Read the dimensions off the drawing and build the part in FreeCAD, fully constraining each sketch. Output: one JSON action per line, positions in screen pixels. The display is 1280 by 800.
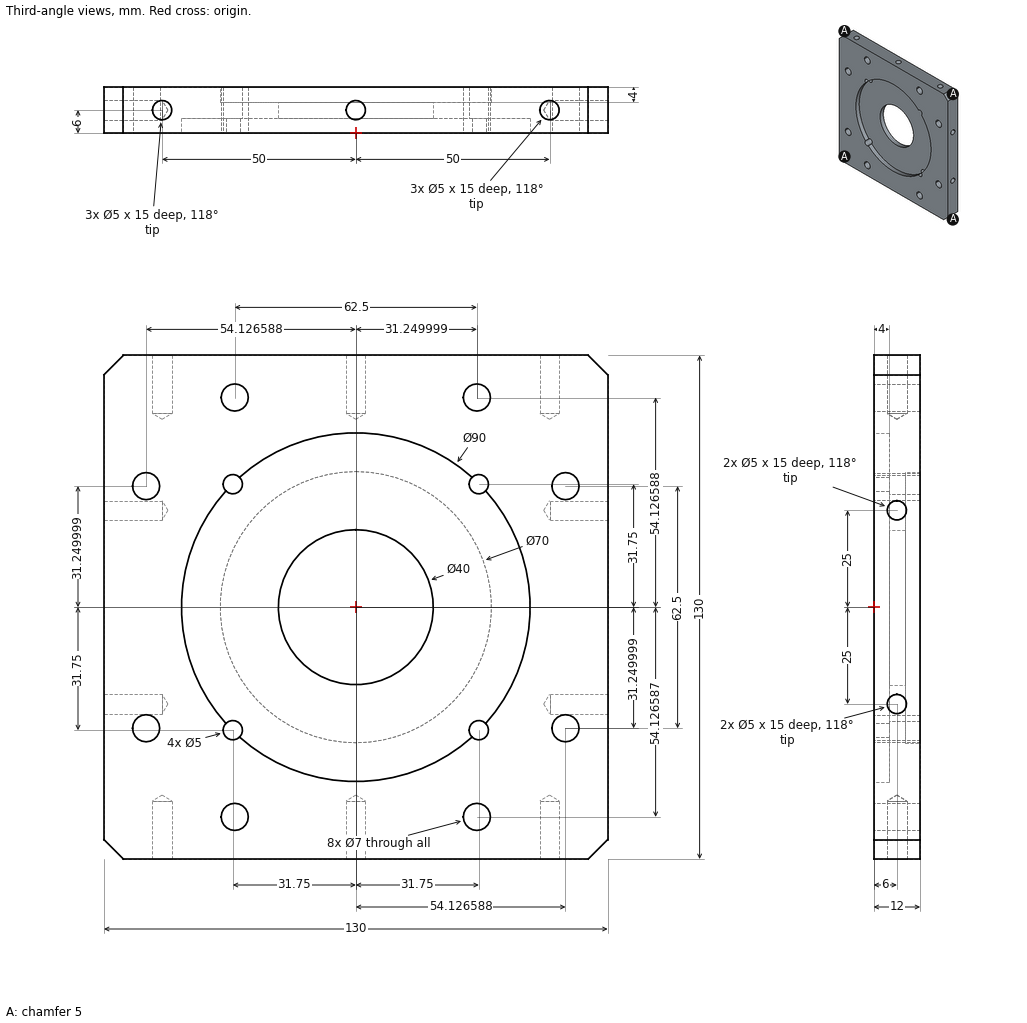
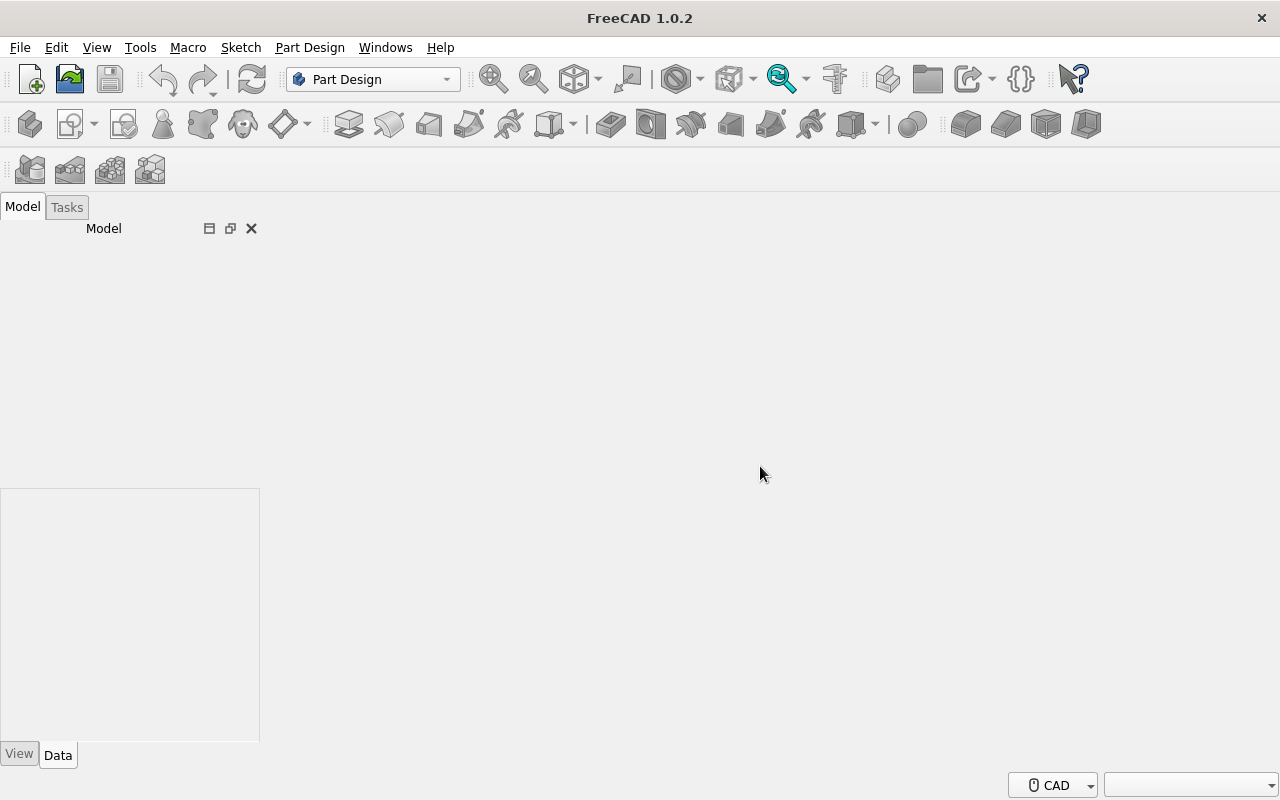
{"action": "key", "text": "ctrl+n"}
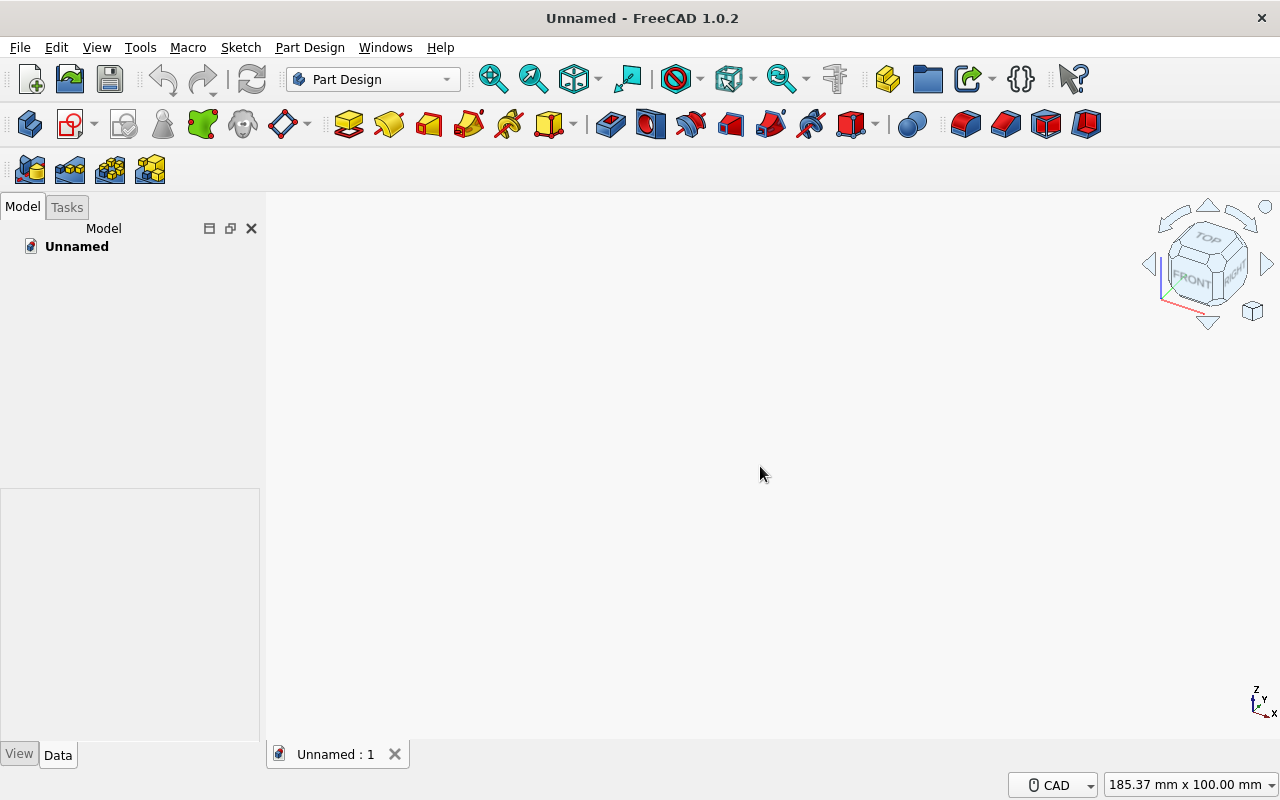
{"action": "left_click", "coordinate": [70, 124]}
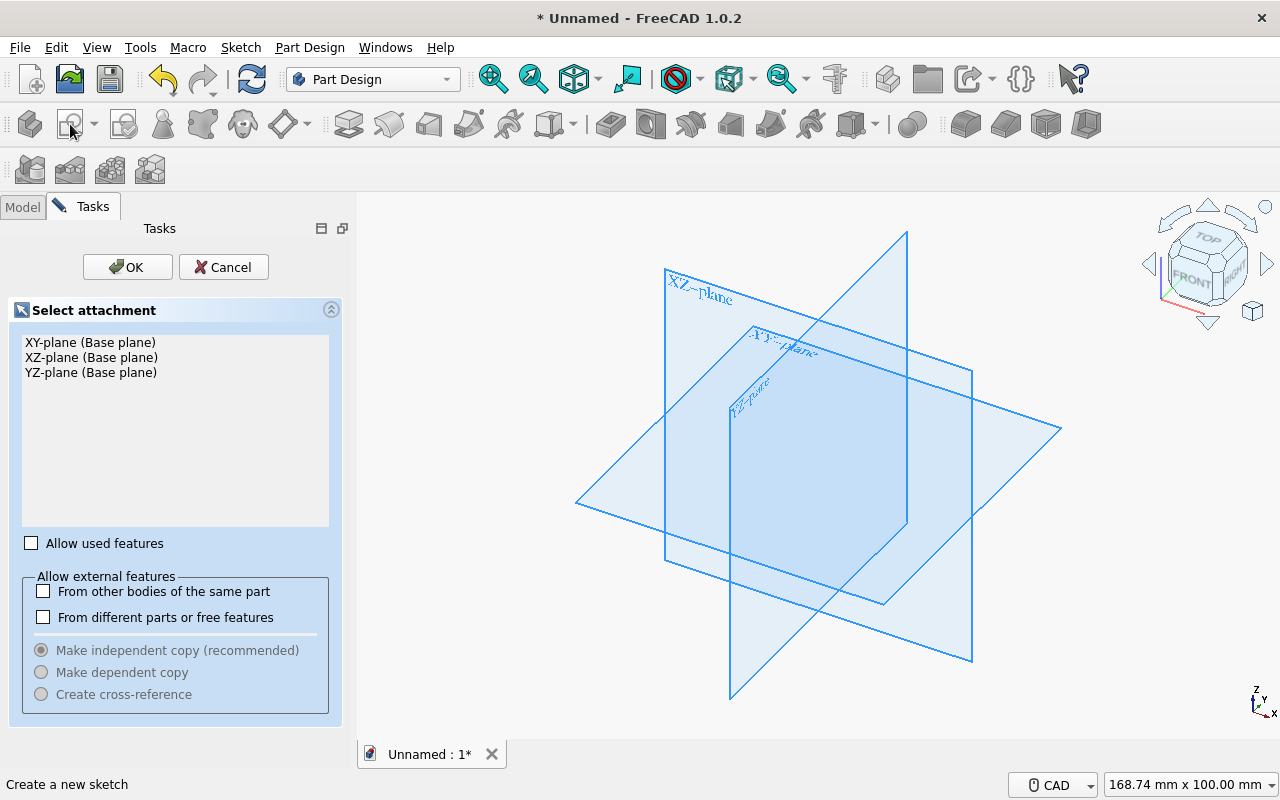
{"action": "left_click", "coordinate": [82, 358]}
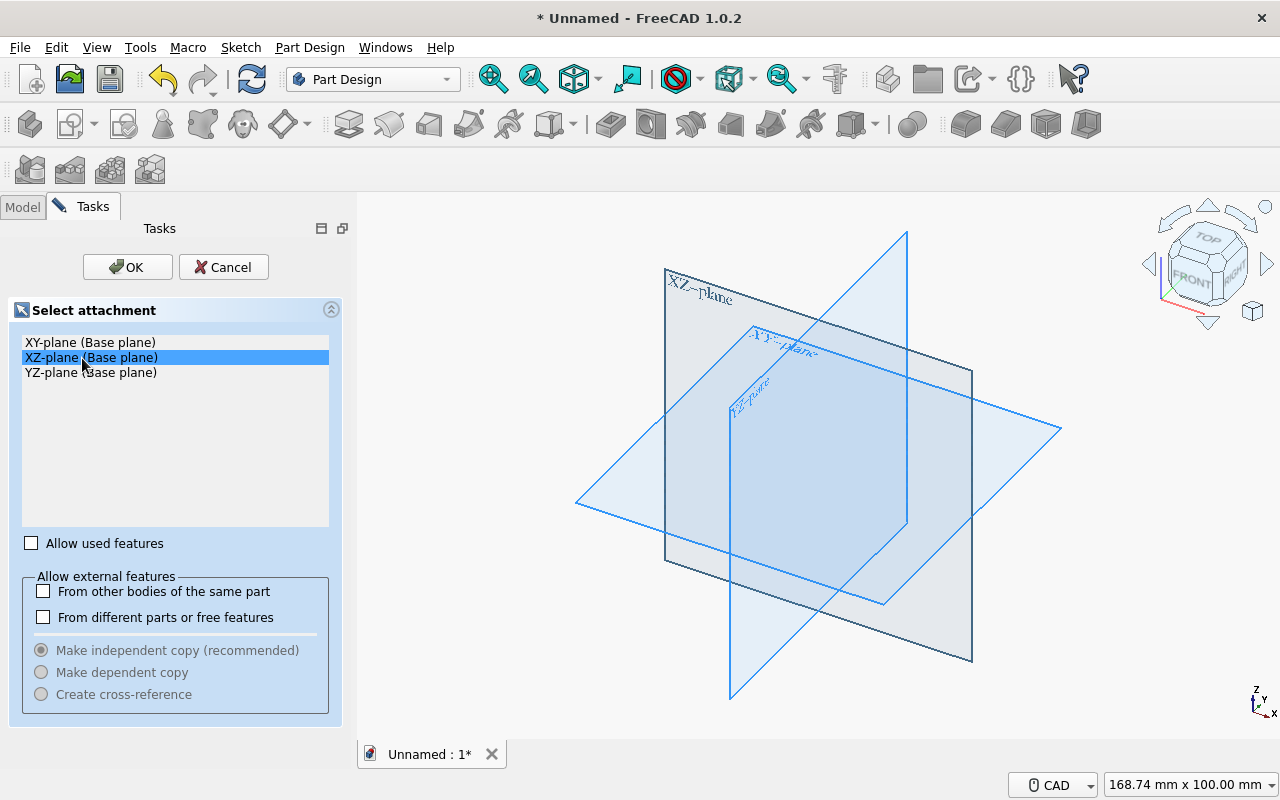
{"action": "left_click", "coordinate": [128, 267]}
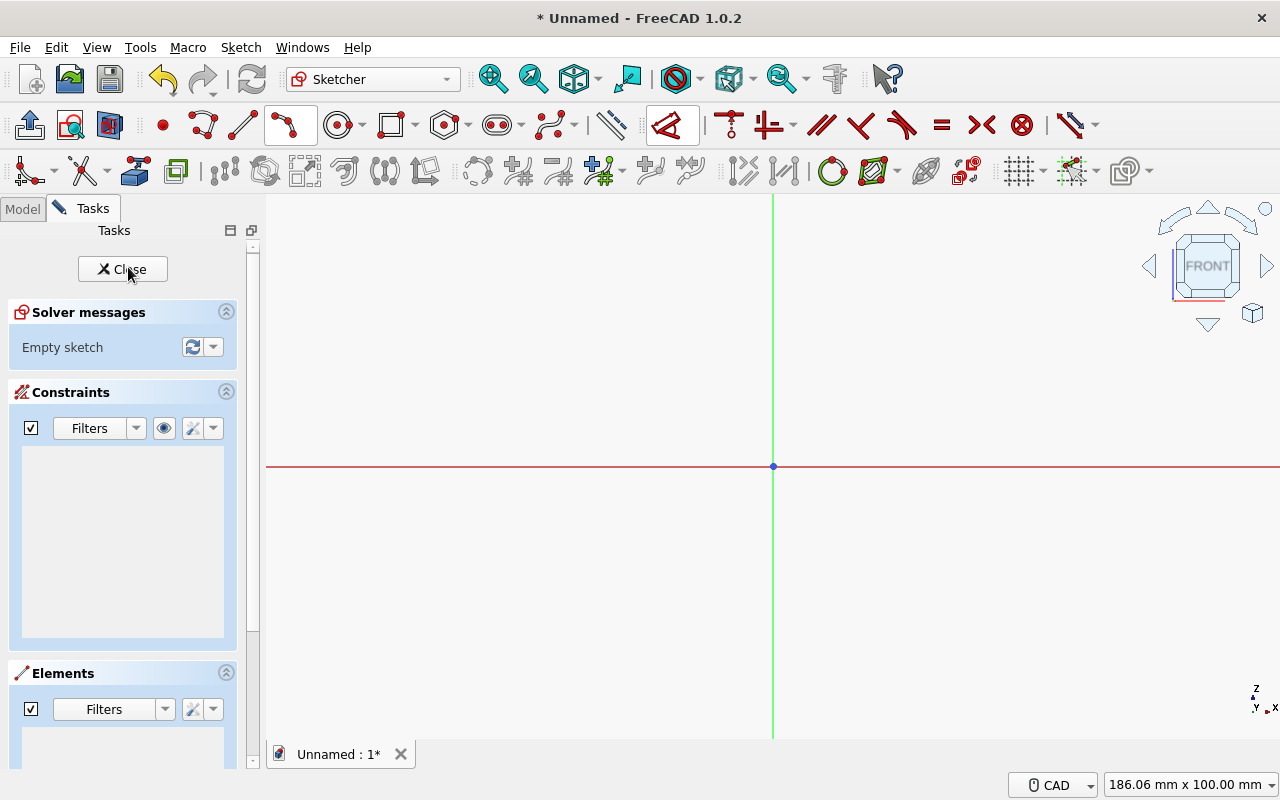
{"action": "scroll", "coordinate": [649, 466], "scroll_direction": "down", "scroll_amount": 4}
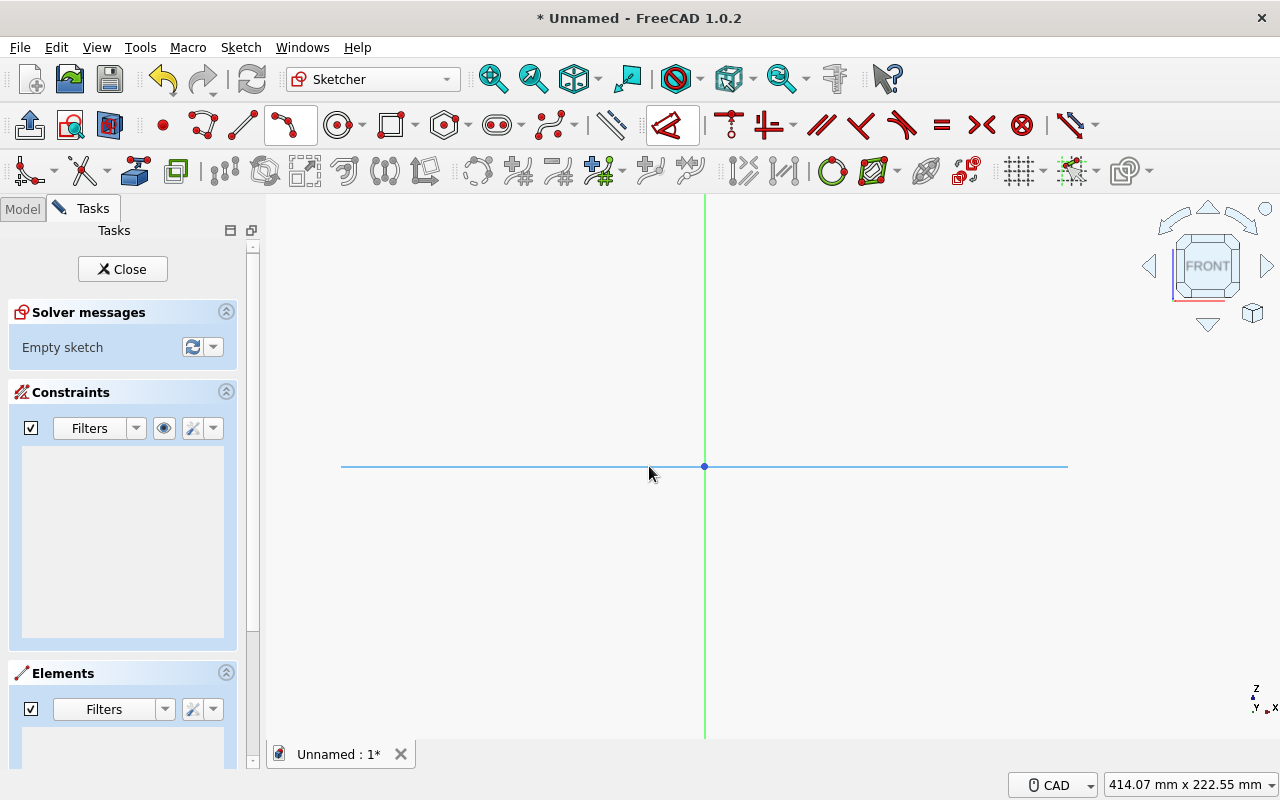
{"action": "key", "text": "g v"}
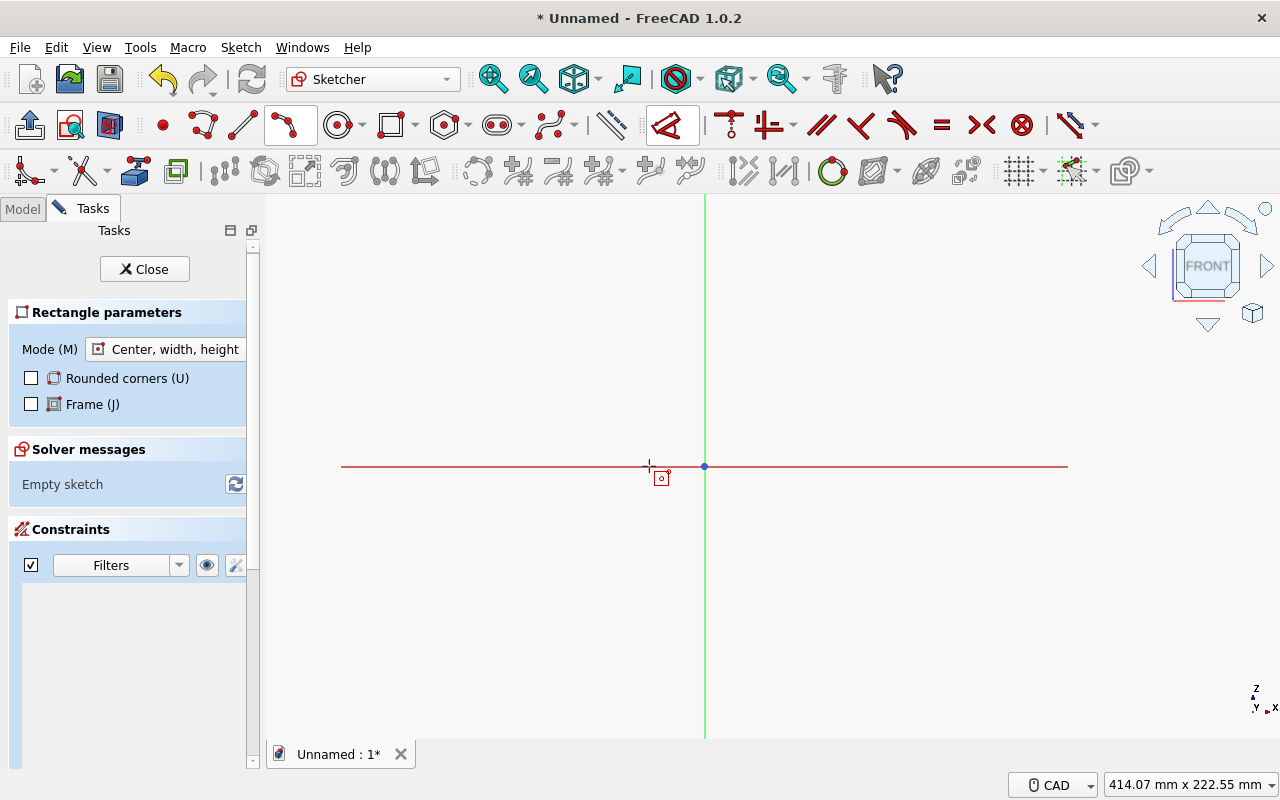
{"action": "left_click", "coordinate": [705, 466]}
{"action": "left_click", "coordinate": [864, 307]}
{"action": "key", "text": "Escape"}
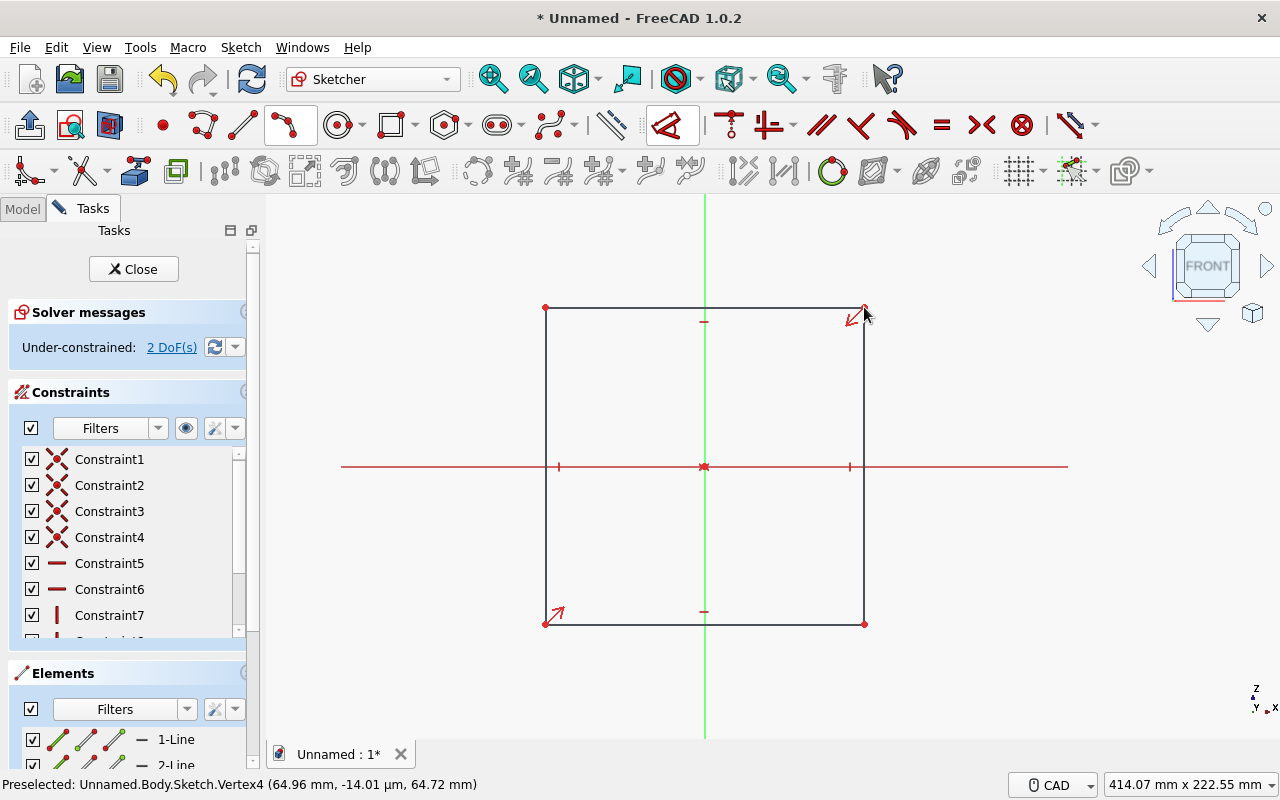
{"action": "key", "text": "d"}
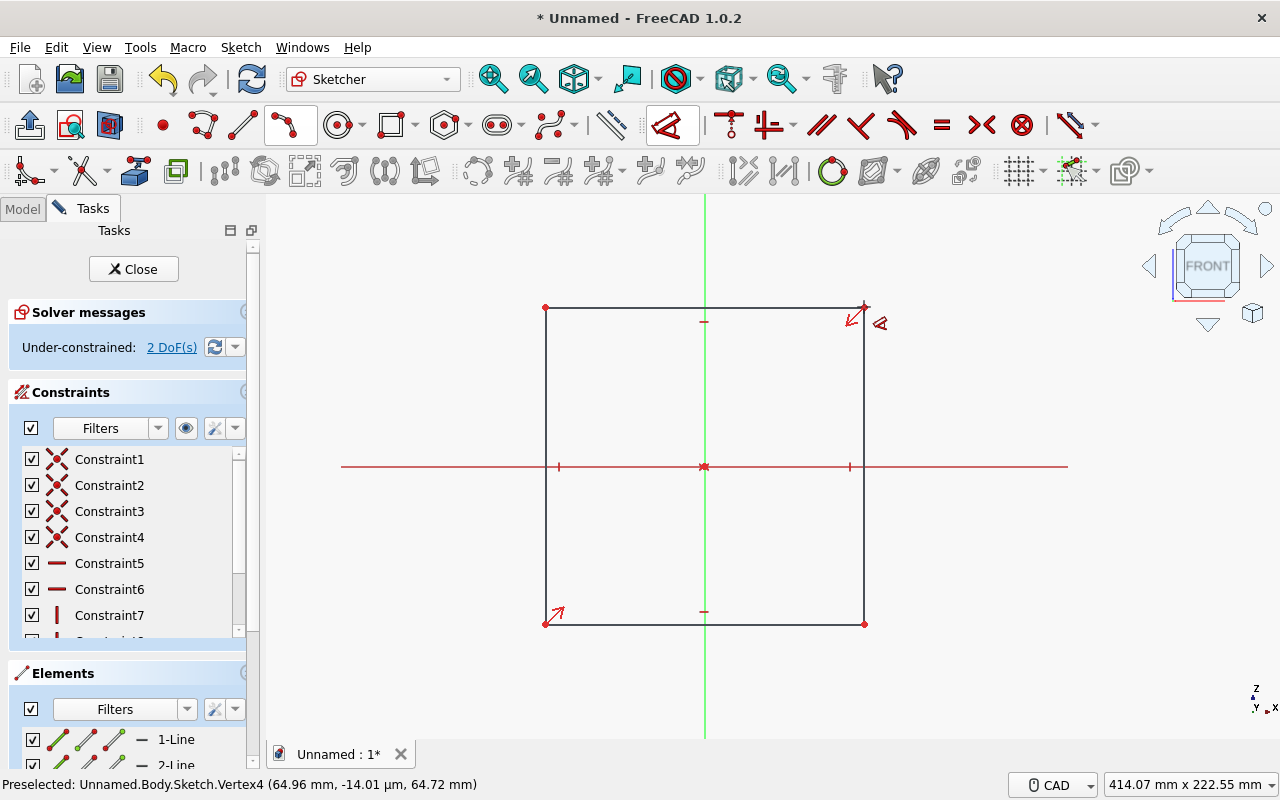
{"action": "left_click", "coordinate": [641, 625]}
{"action": "left_click", "coordinate": [632, 659]}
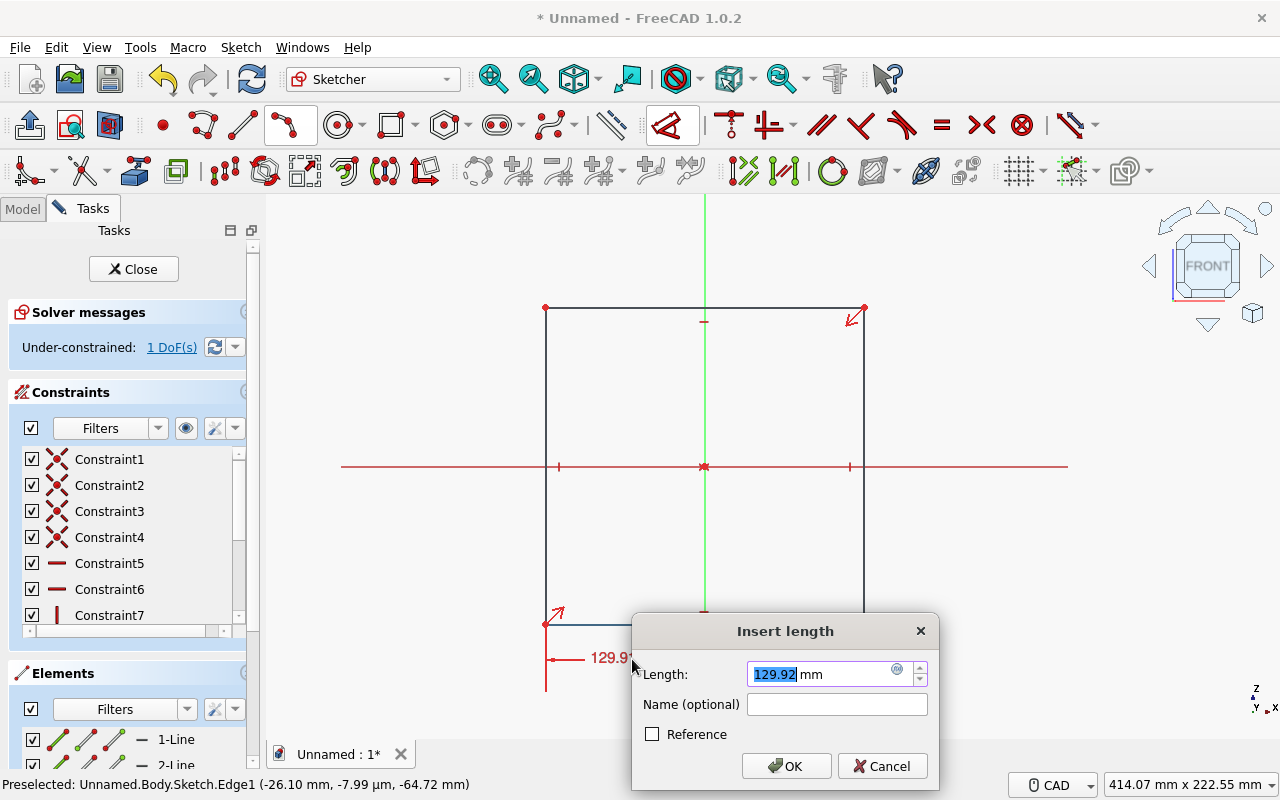
{"action": "type", "text": "130"}
{"action": "key", "text": "Return"}